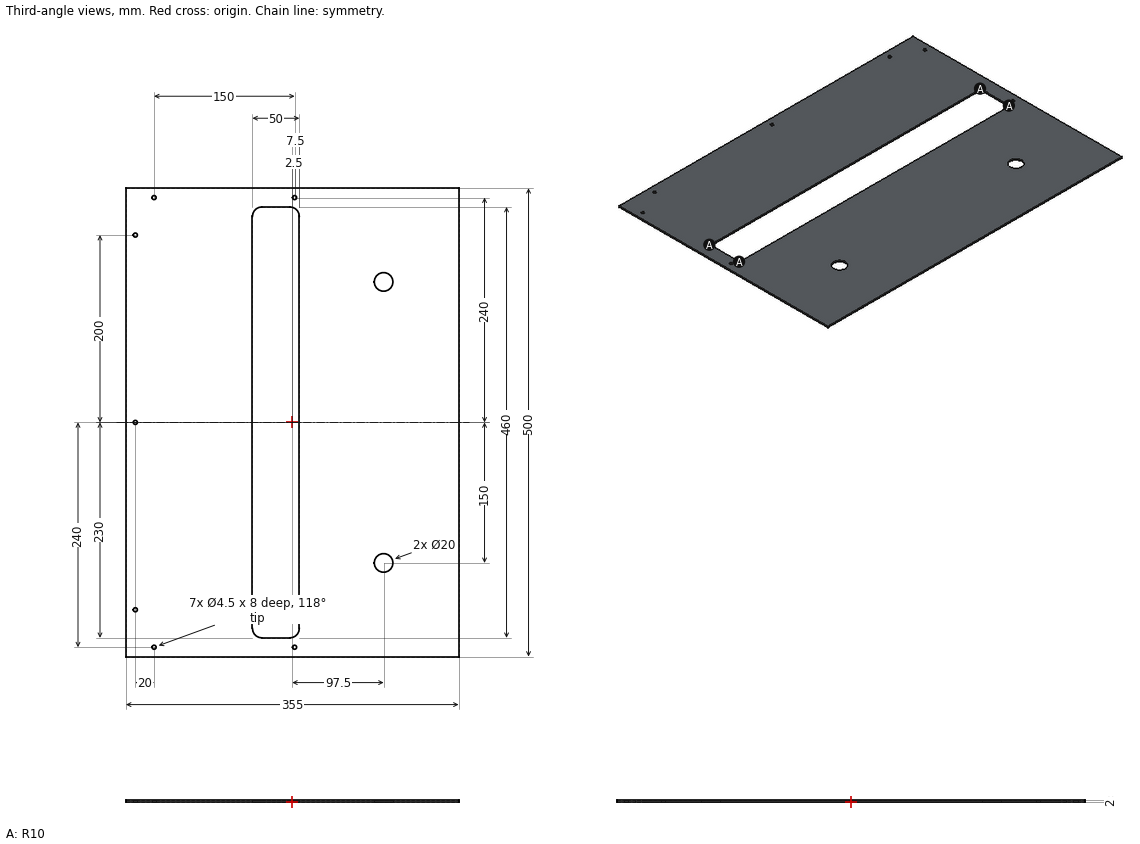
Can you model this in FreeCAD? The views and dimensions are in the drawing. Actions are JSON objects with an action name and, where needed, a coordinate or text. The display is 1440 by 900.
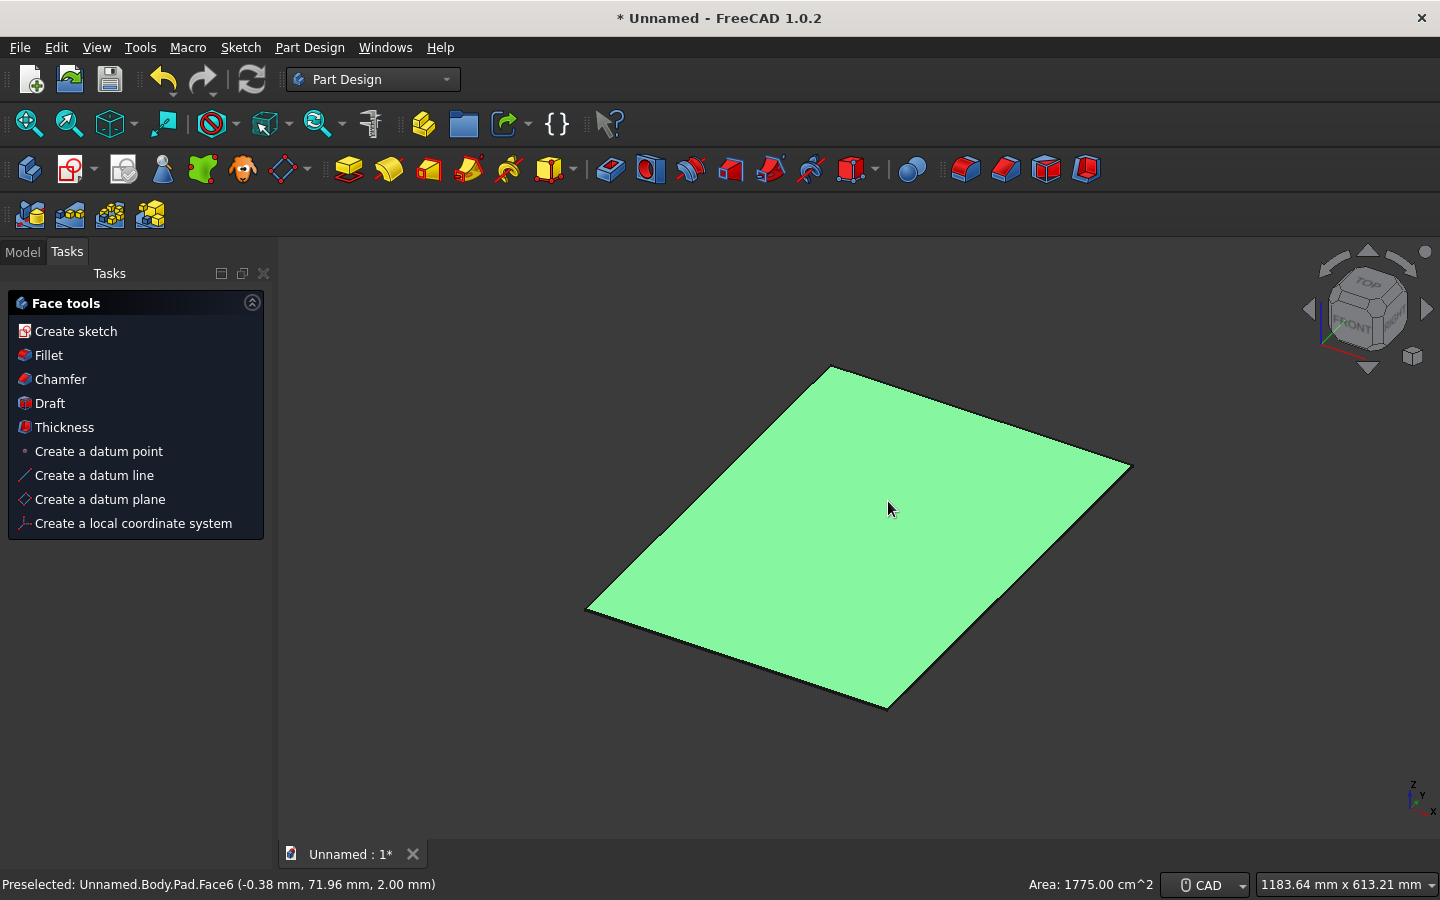
{"action": "left_click", "coordinate": [70, 170]}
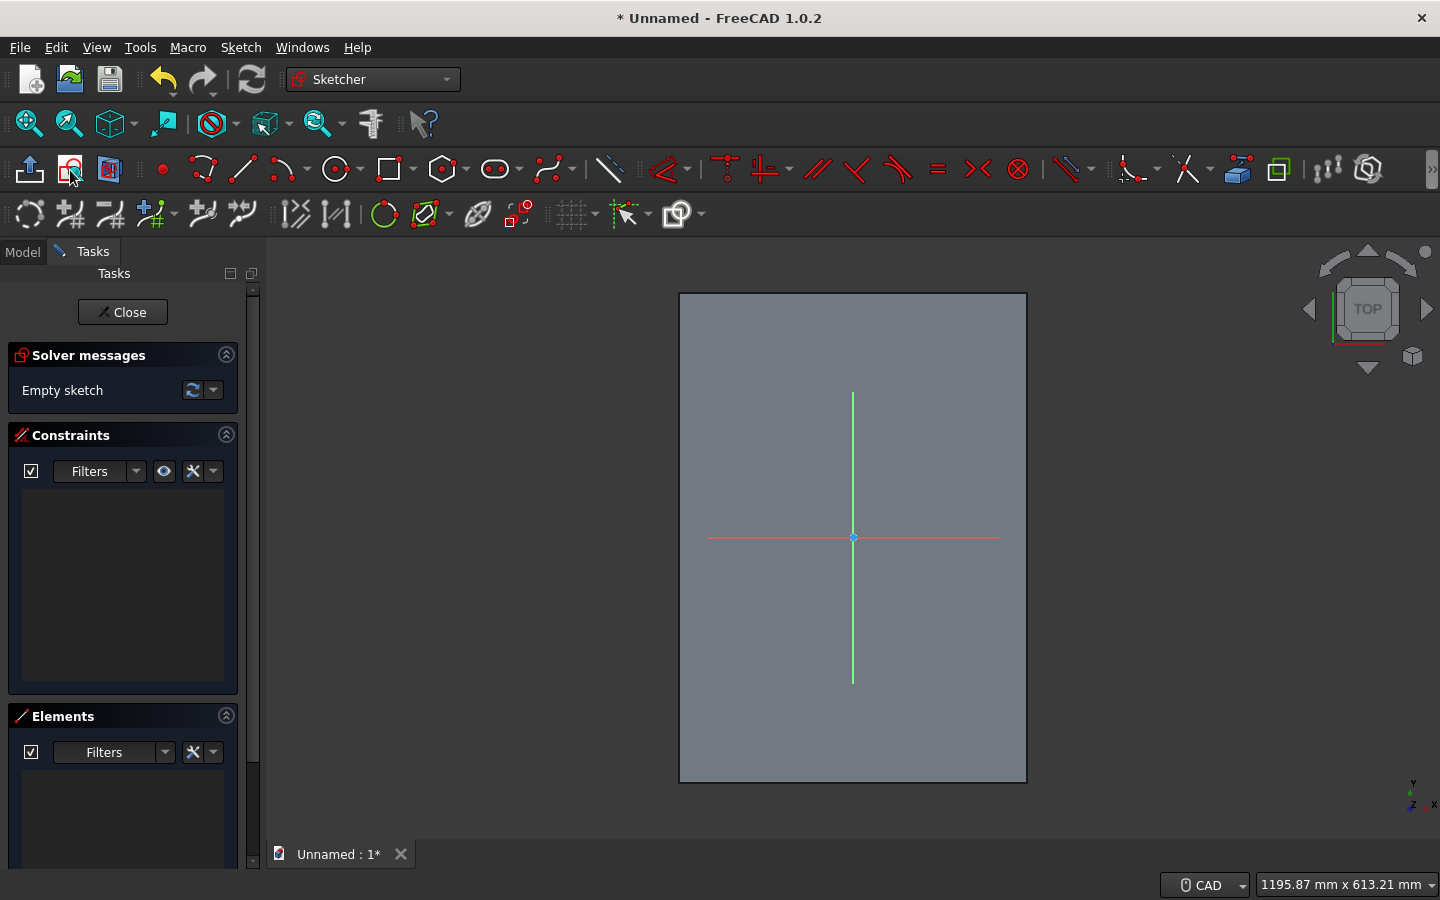
{"action": "key", "text": "g c"}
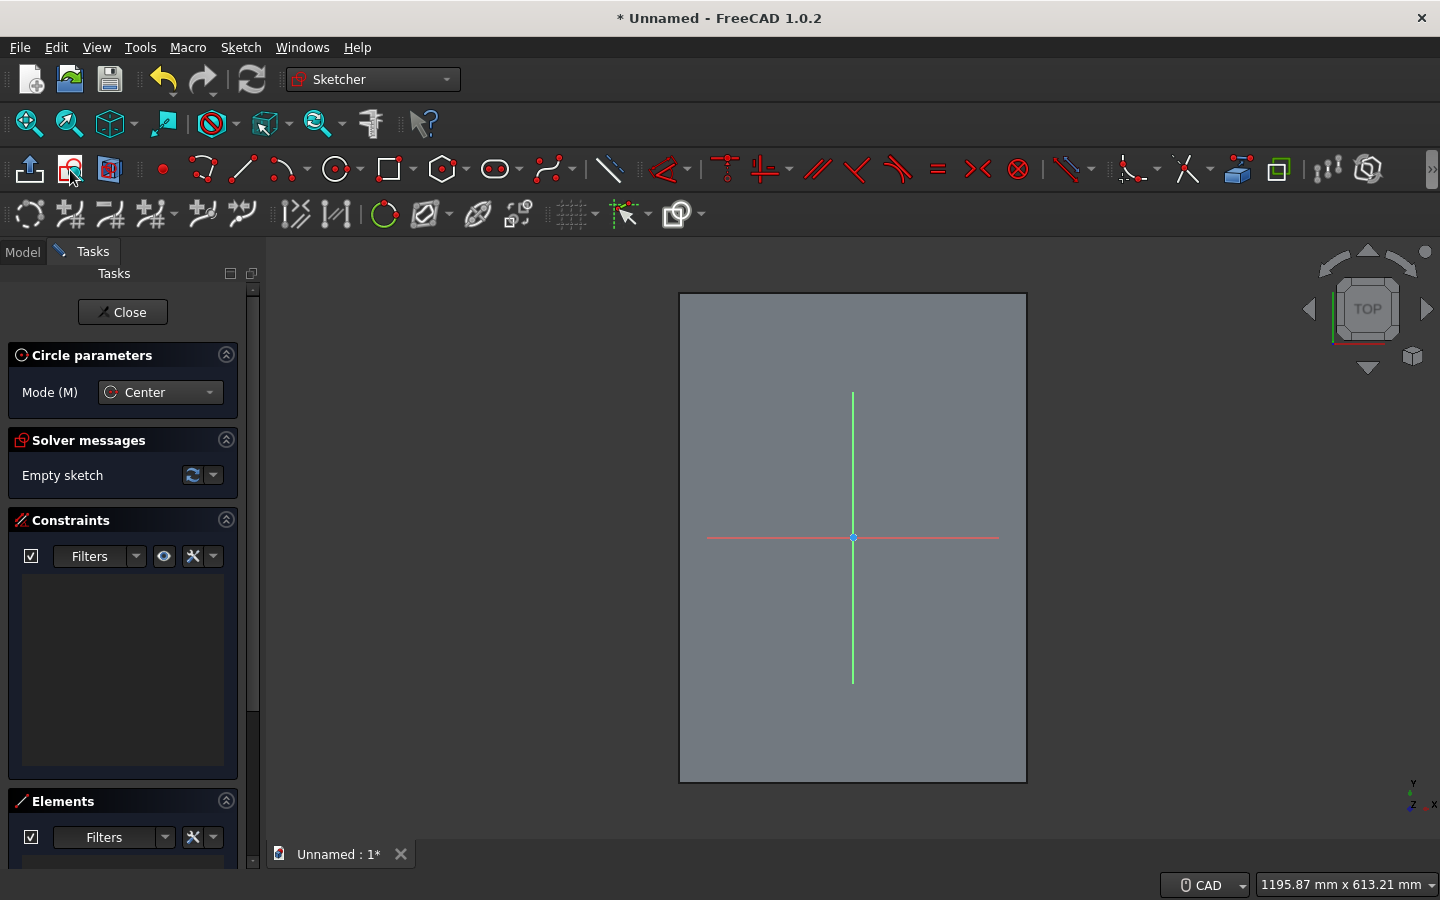
{"action": "scroll", "coordinate": [708, 774], "scroll_direction": "up", "scroll_amount": 12}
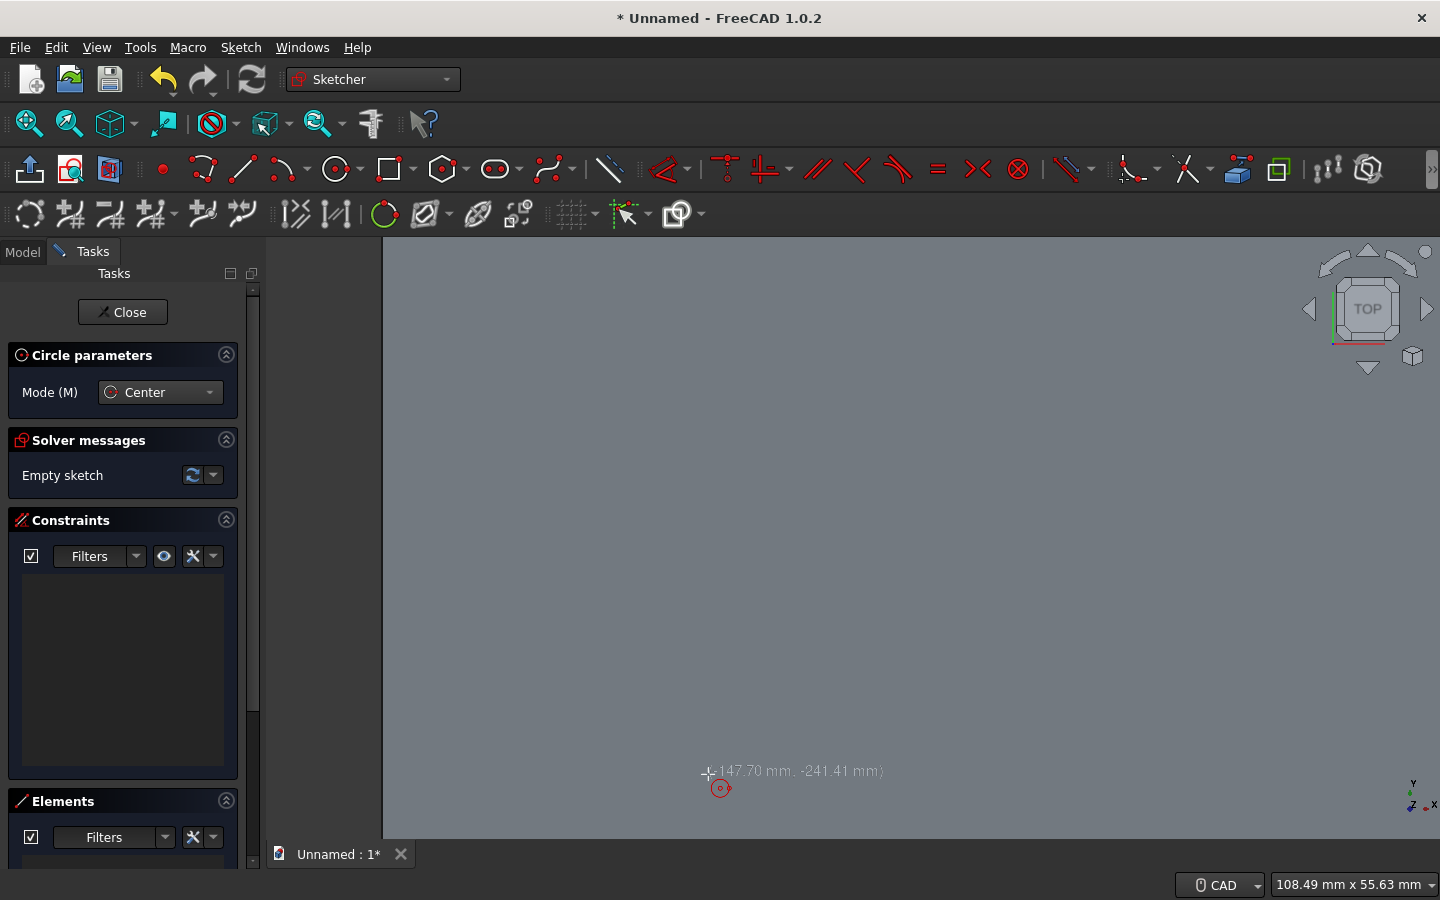
{"action": "scroll", "coordinate": [734, 729], "scroll_direction": "down", "scroll_amount": 13}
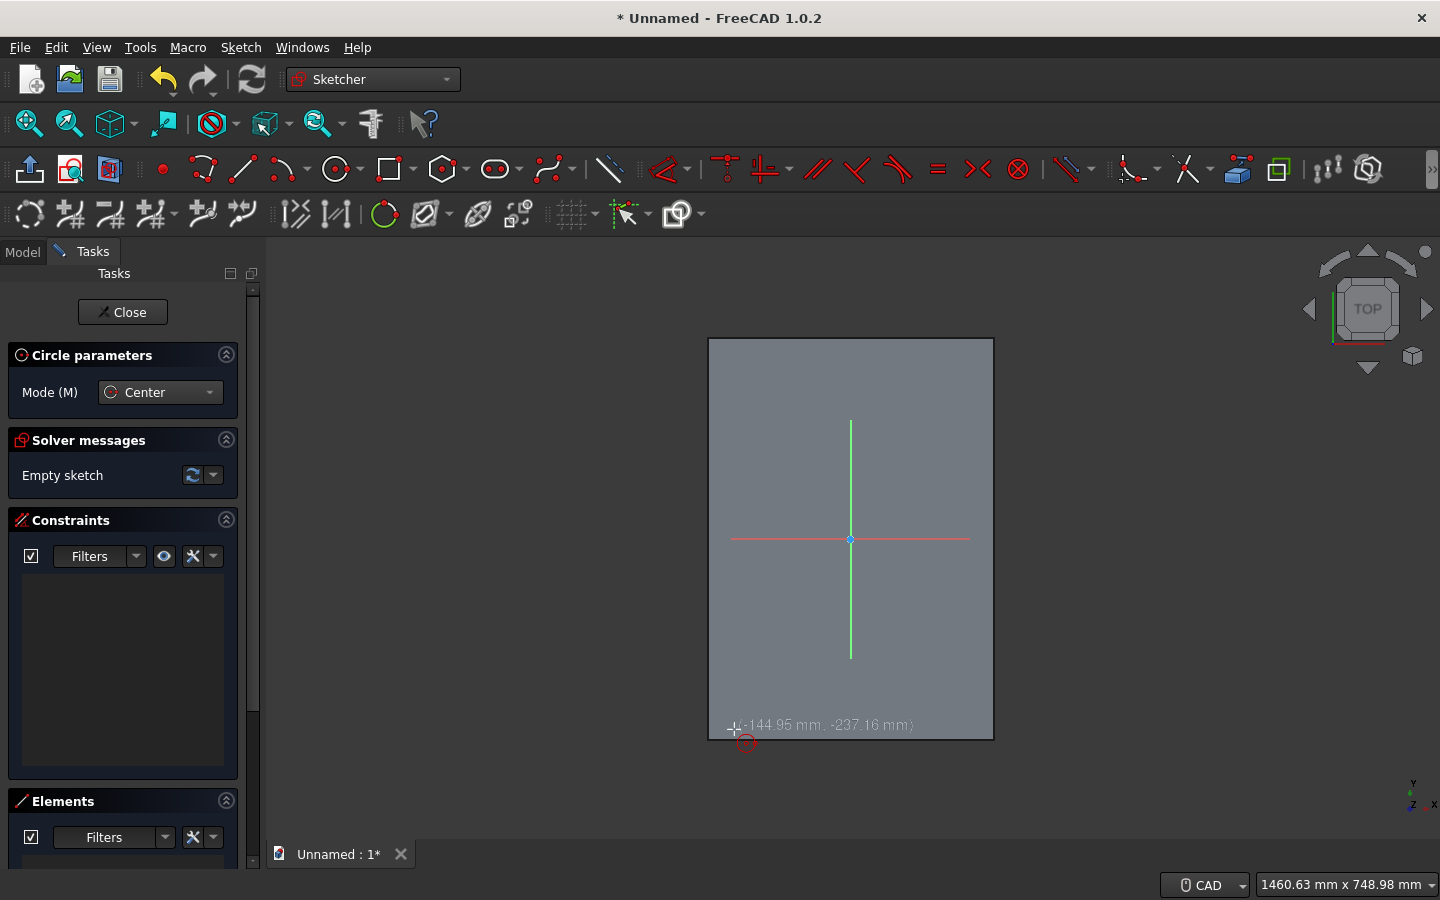
{"action": "left_click", "coordinate": [732, 732]}
{"action": "mouse_move", "coordinate": [734, 731]}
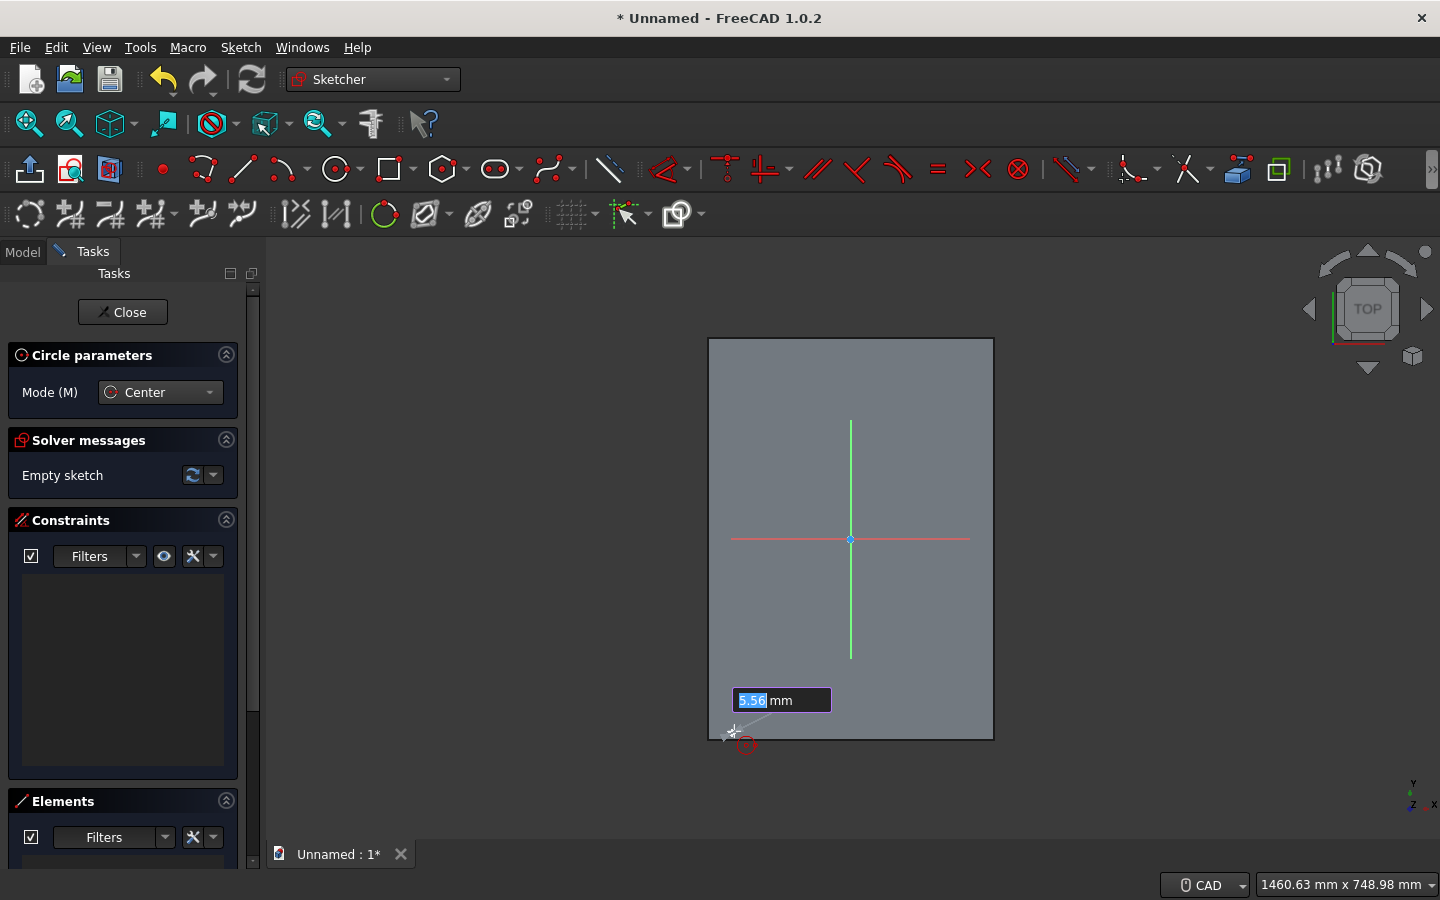
{"action": "type", "text": "4.5"}
{"action": "key", "text": "Return"}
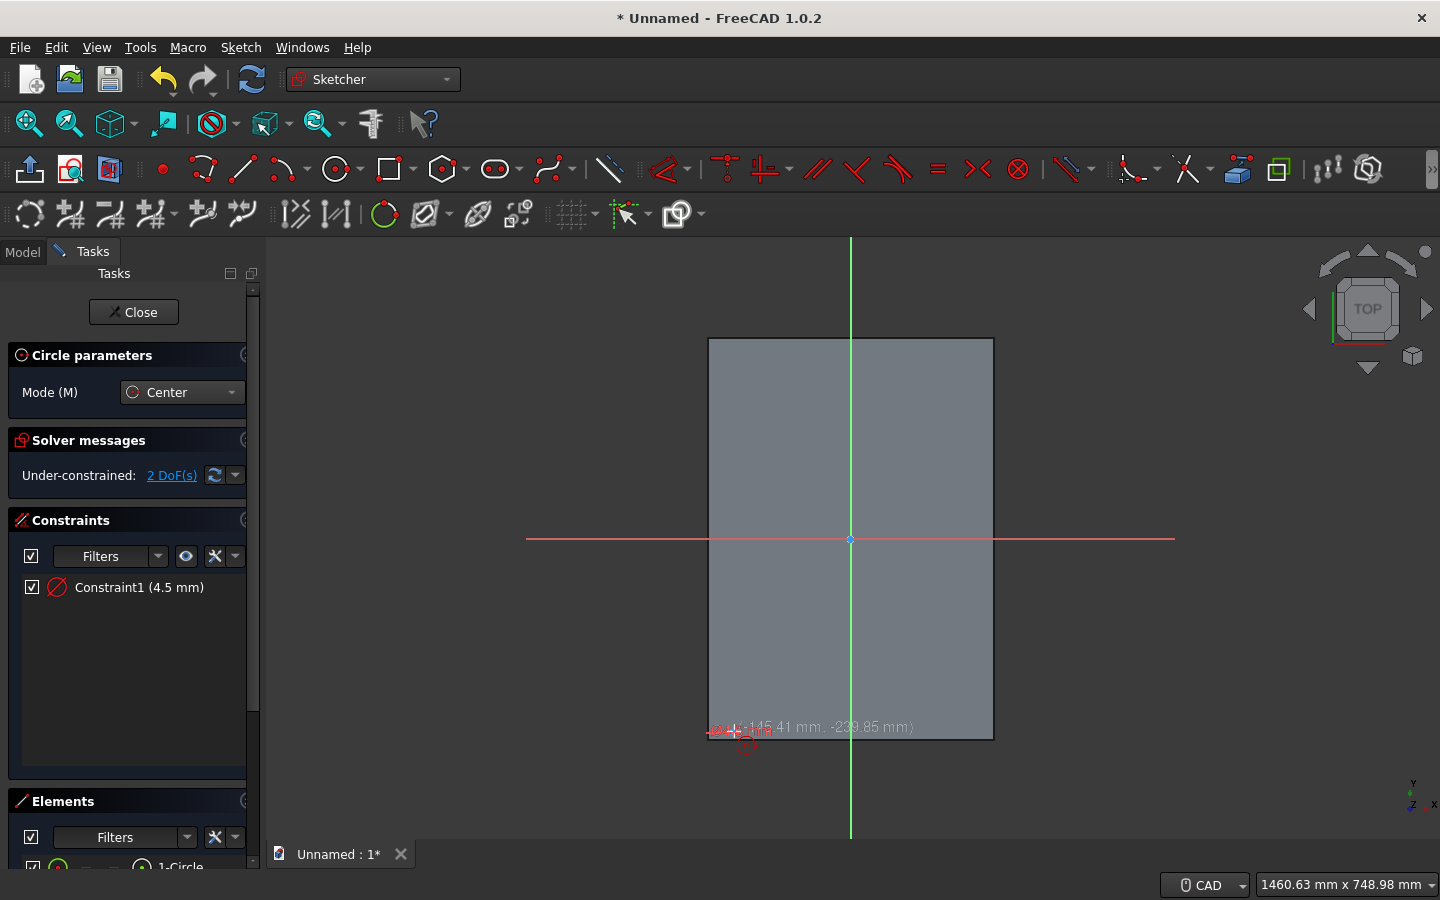
{"action": "scroll", "coordinate": [716, 539], "scroll_direction": "up", "scroll_amount": 13}